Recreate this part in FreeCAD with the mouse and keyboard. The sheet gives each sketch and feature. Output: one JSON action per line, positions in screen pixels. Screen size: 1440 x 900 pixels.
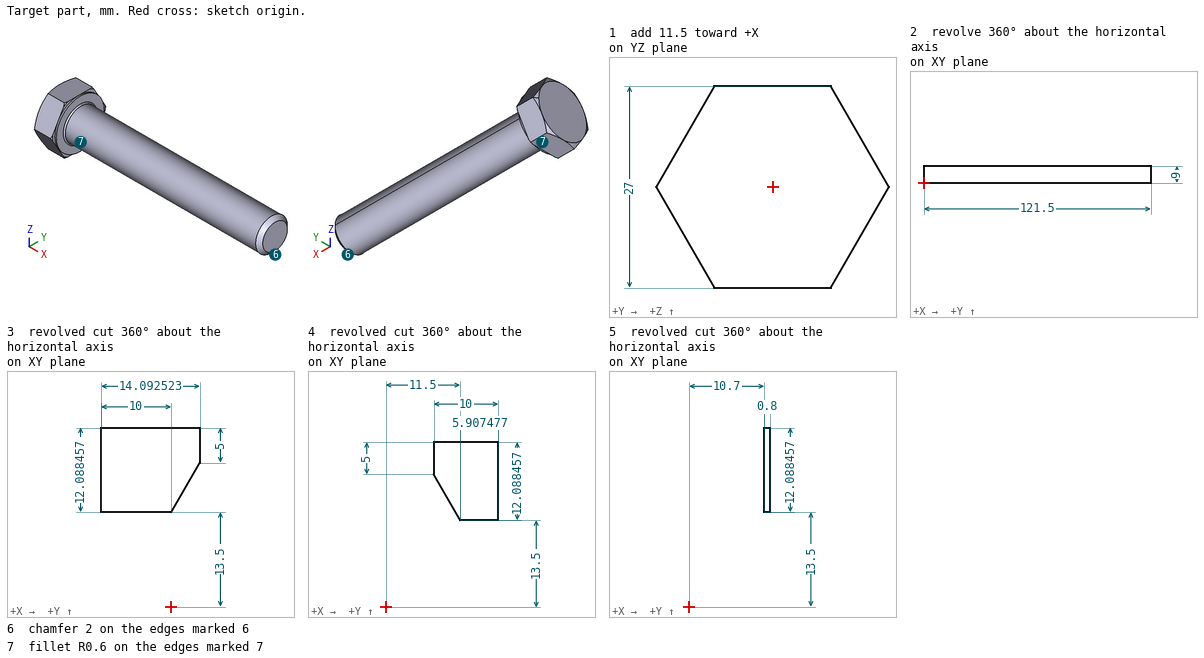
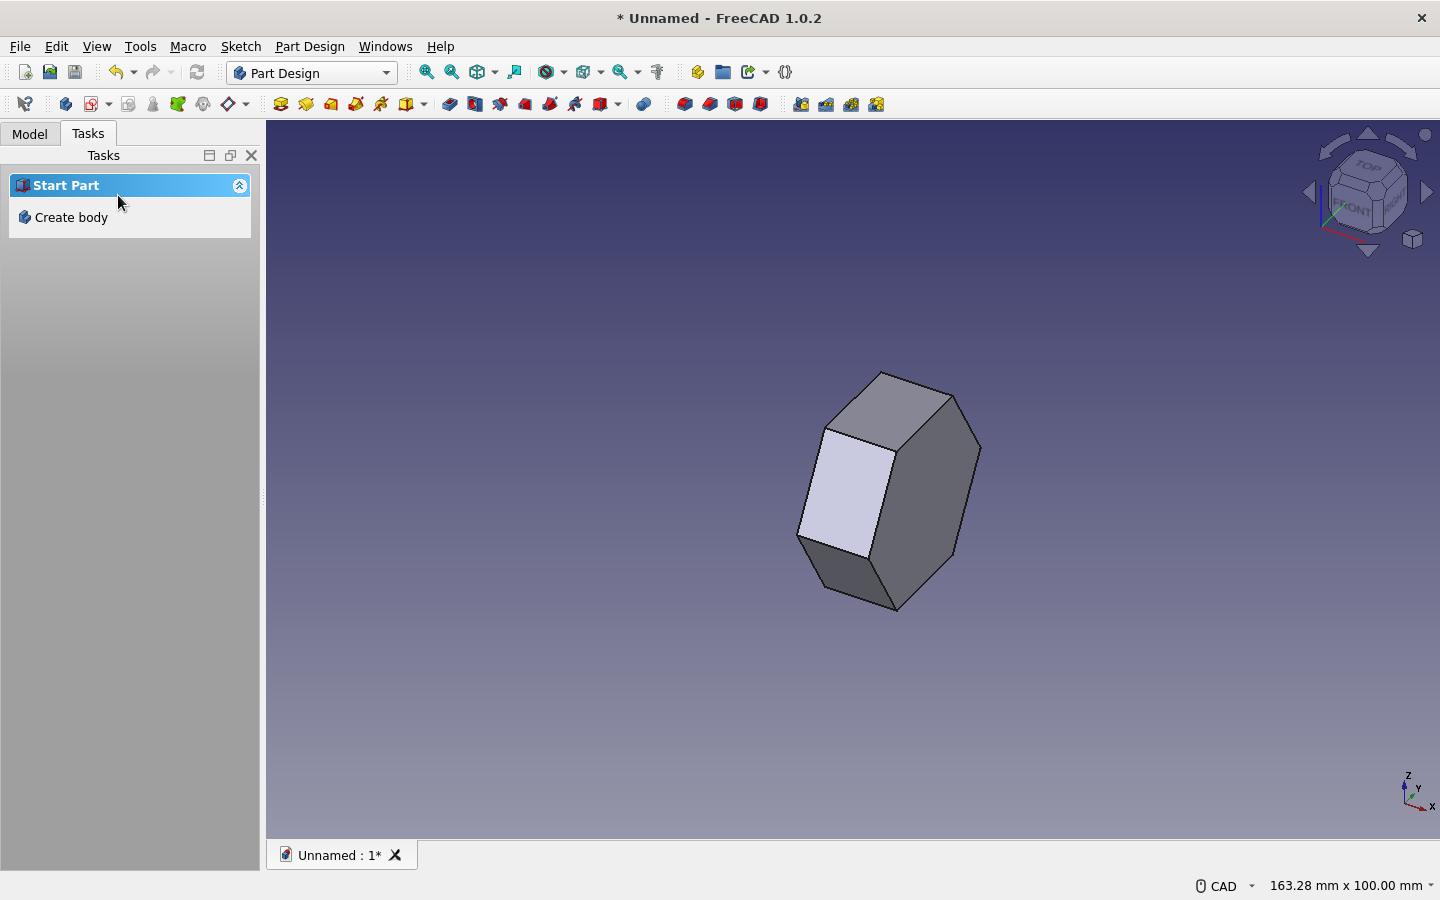
{"action": "left_click", "coordinate": [427, 72]}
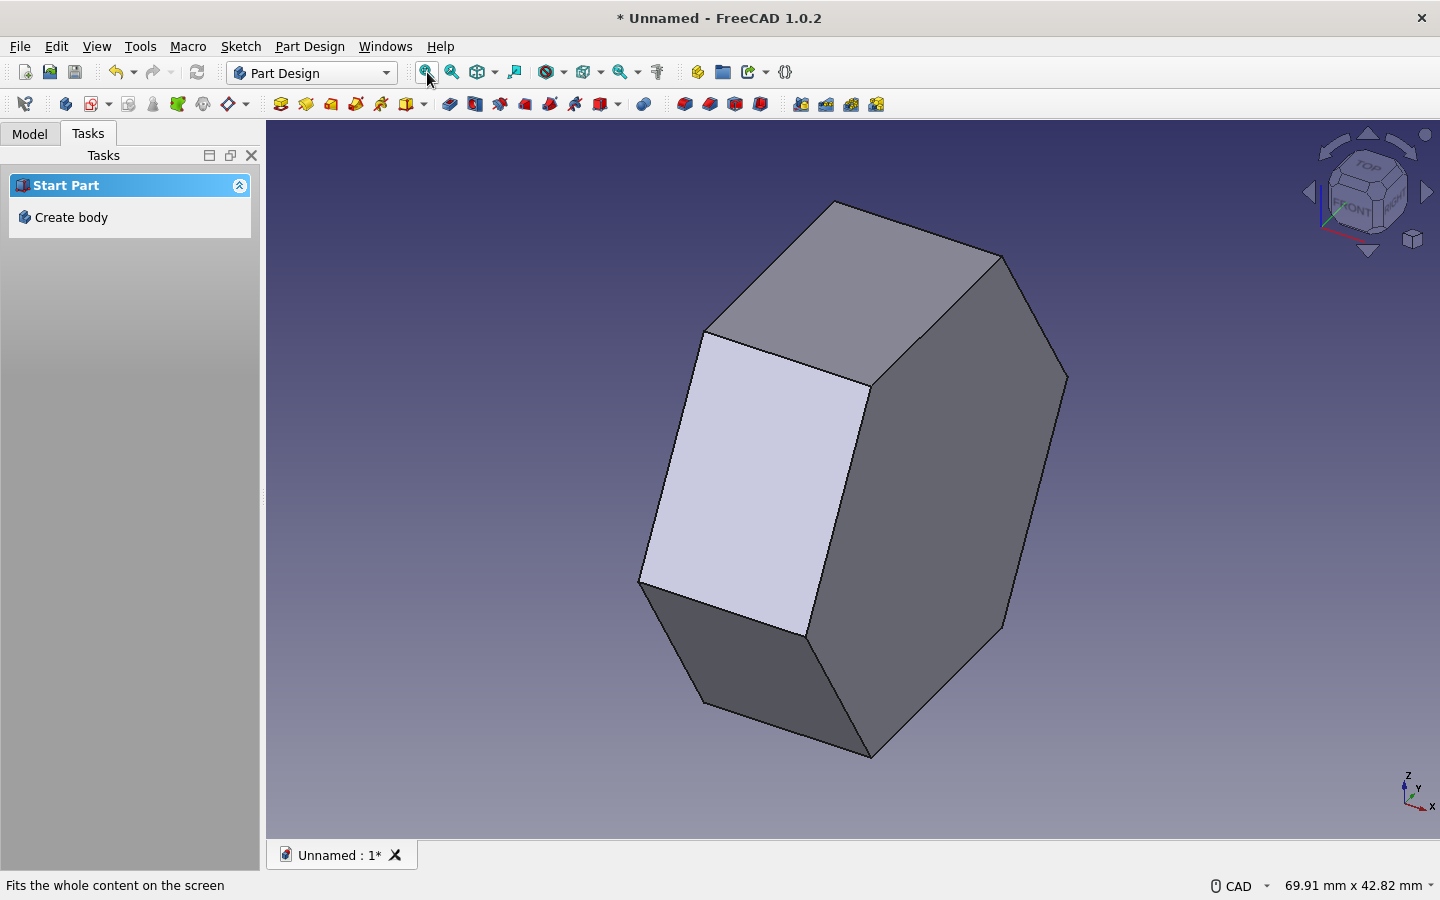
{"action": "left_click", "coordinate": [90, 104]}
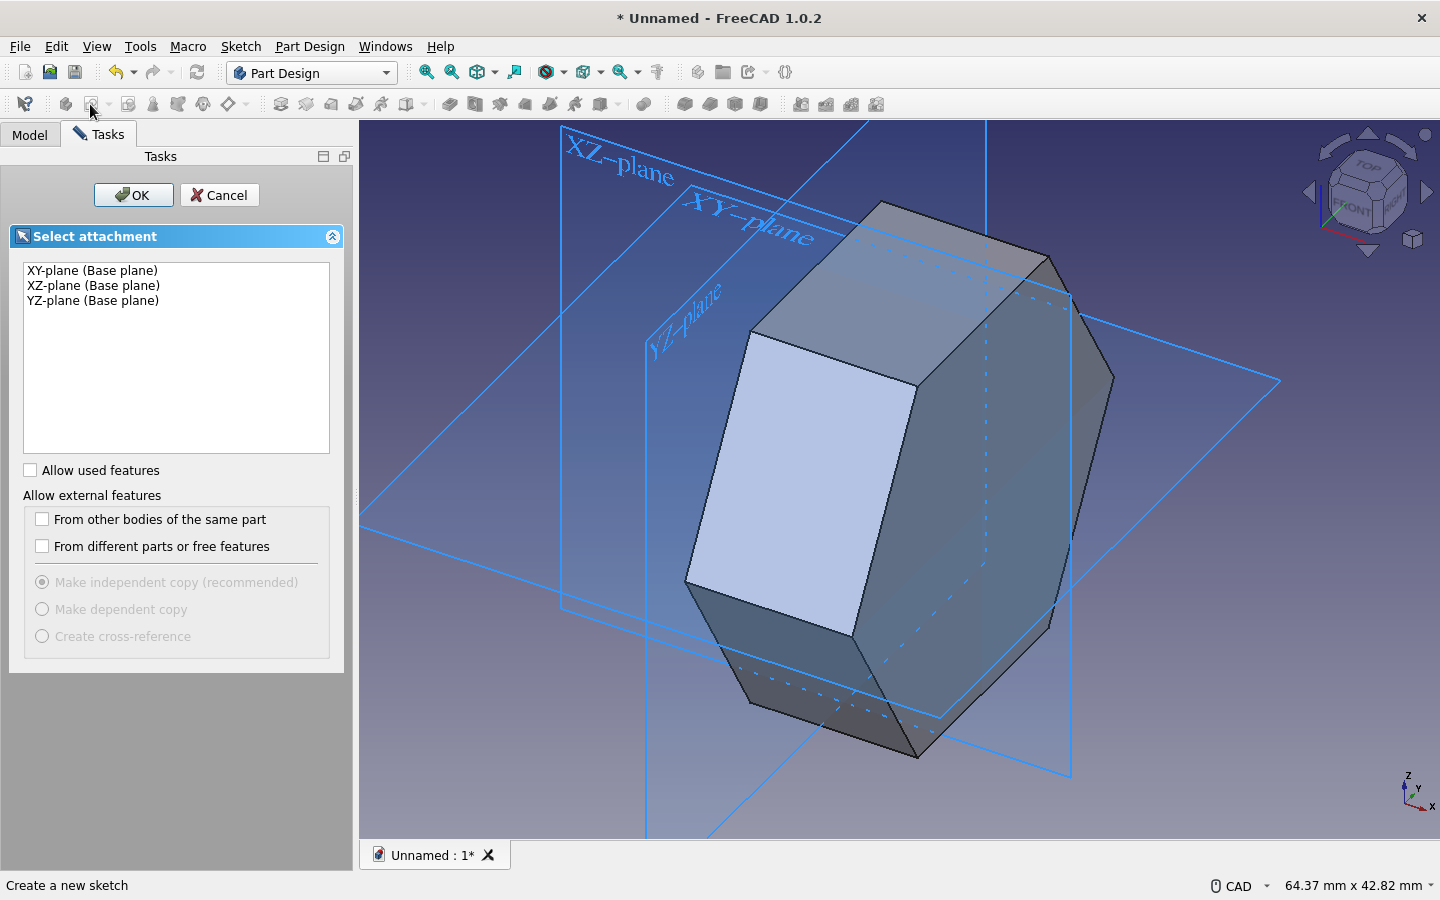
{"action": "left_click", "coordinate": [84, 270]}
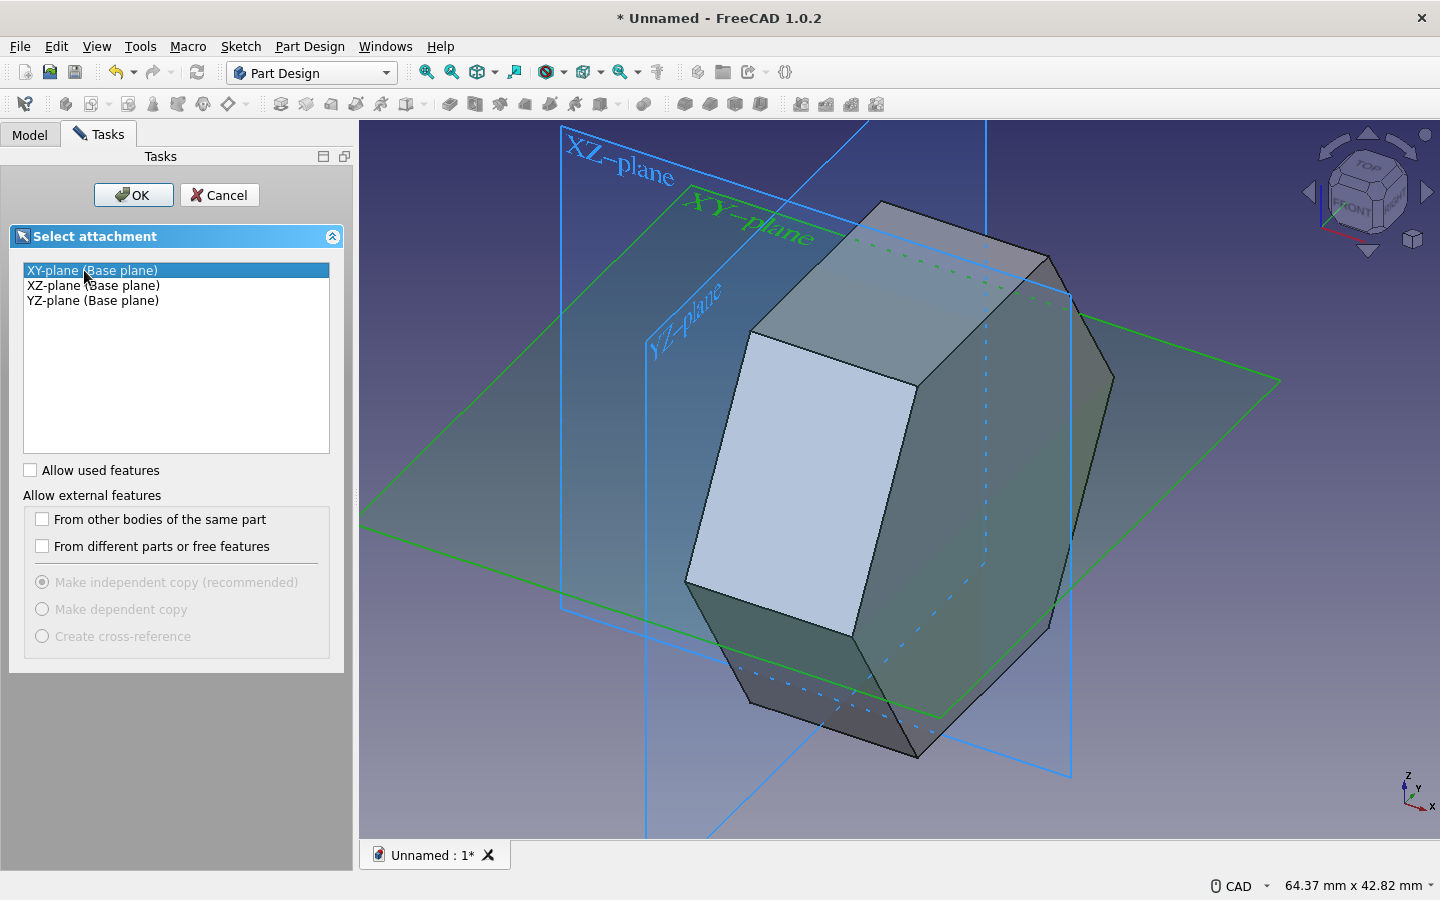
{"action": "left_click", "coordinate": [134, 195]}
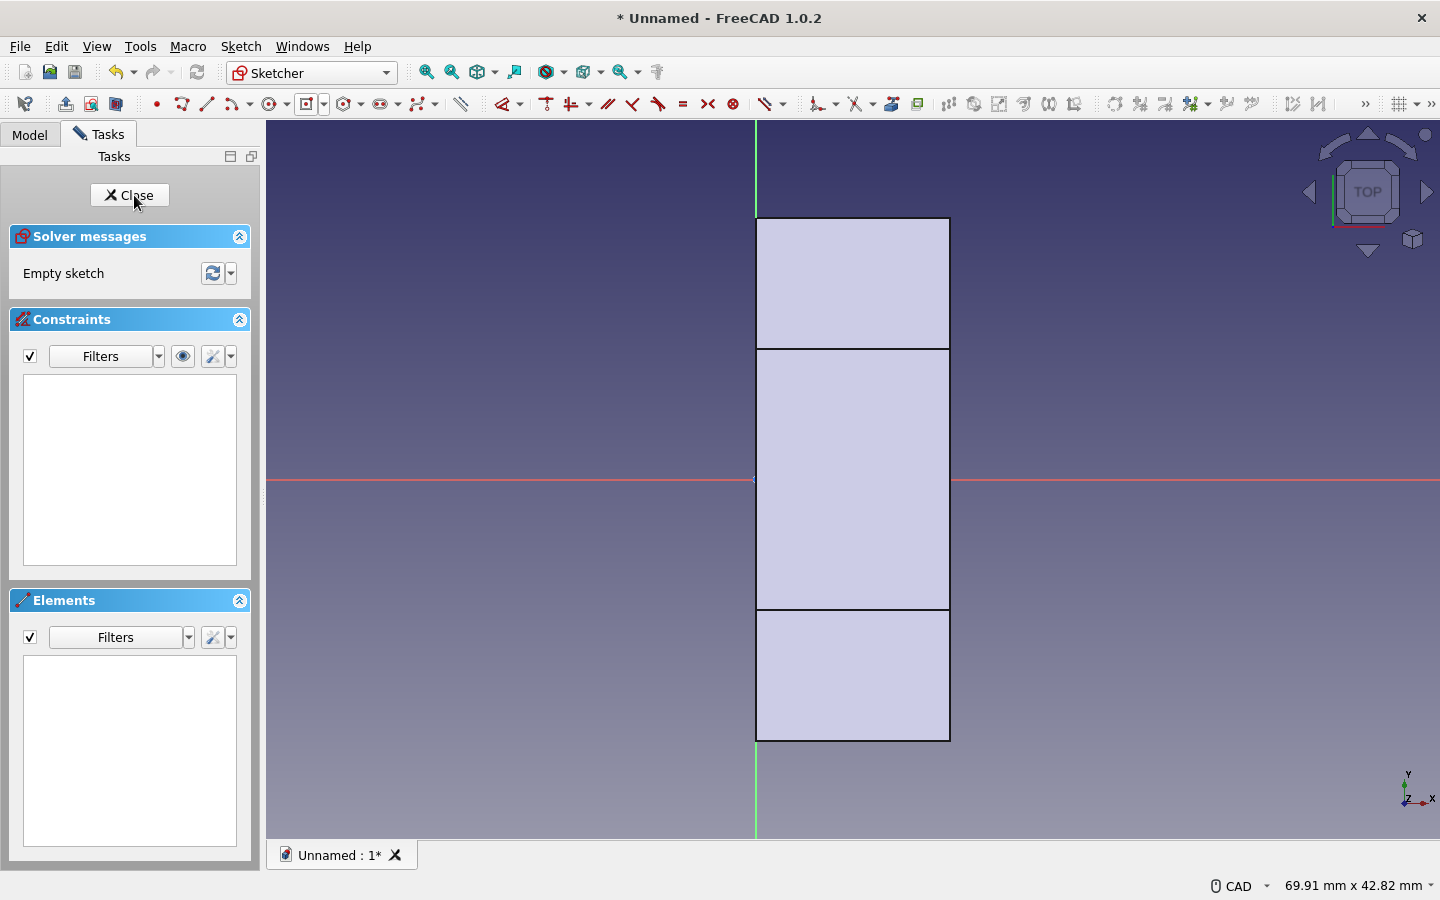
{"action": "left_click", "coordinate": [116, 104]}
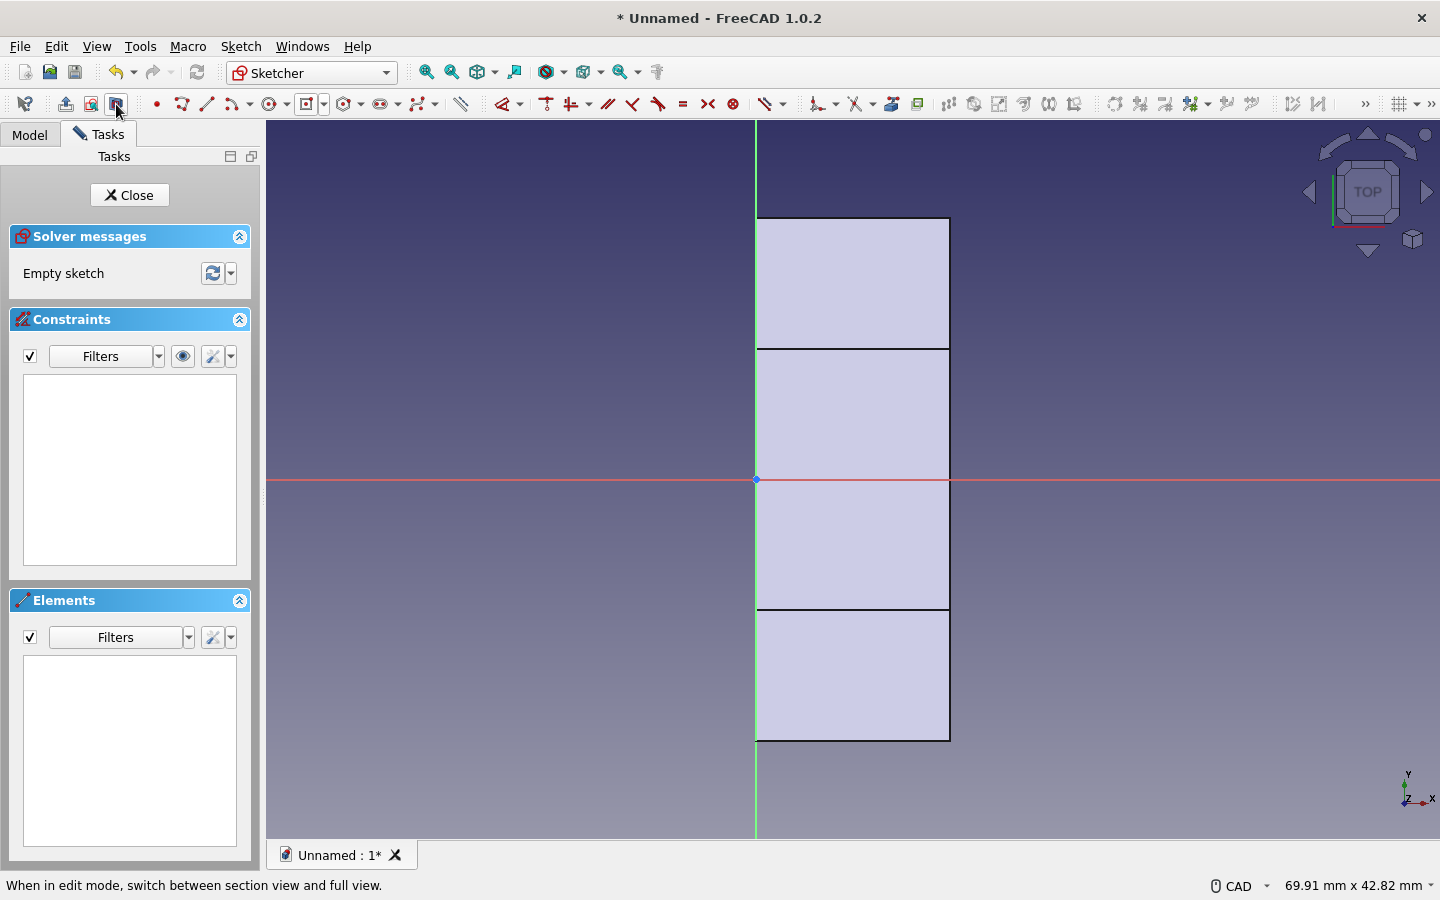
{"action": "scroll", "coordinate": [294, 523], "scroll_direction": "down", "scroll_amount": 5}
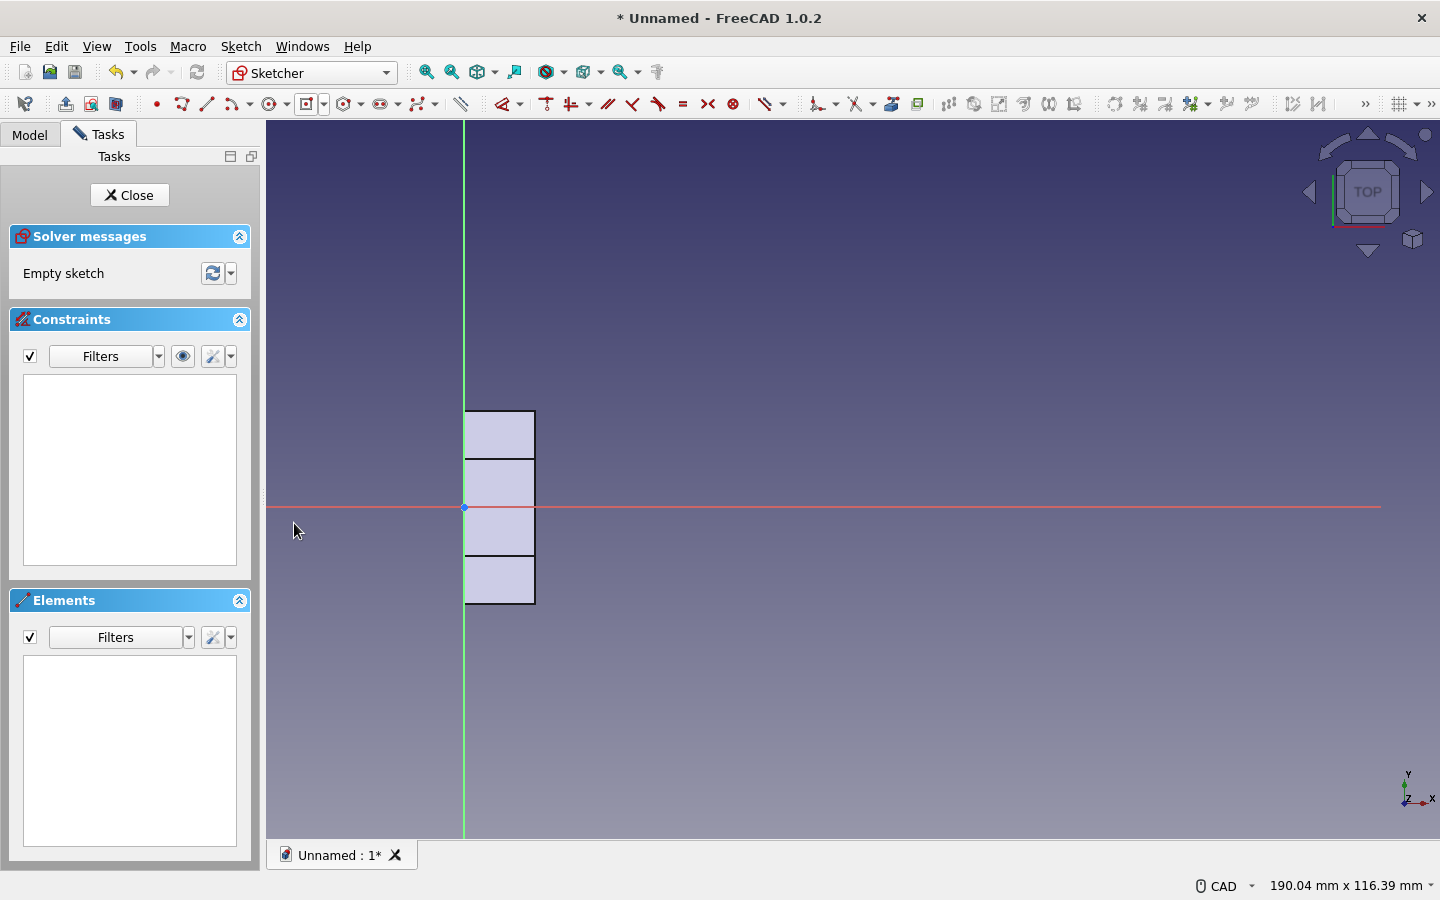
{"action": "key", "text": "g r"}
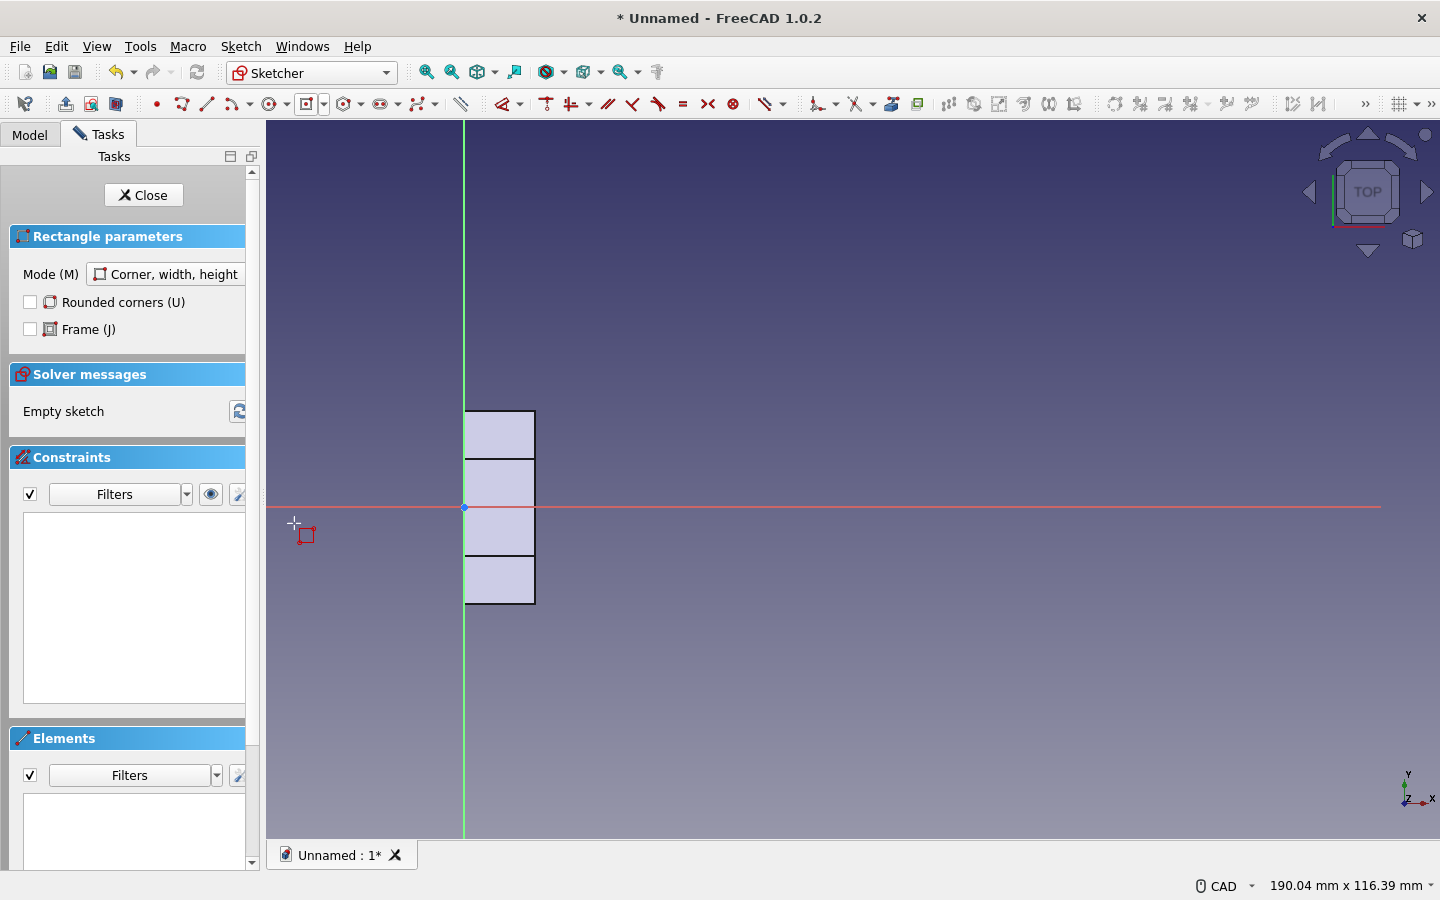
{"action": "left_click", "coordinate": [464, 507]}
{"action": "left_click", "coordinate": [1215, 452]}
{"action": "key", "text": "Escape"}